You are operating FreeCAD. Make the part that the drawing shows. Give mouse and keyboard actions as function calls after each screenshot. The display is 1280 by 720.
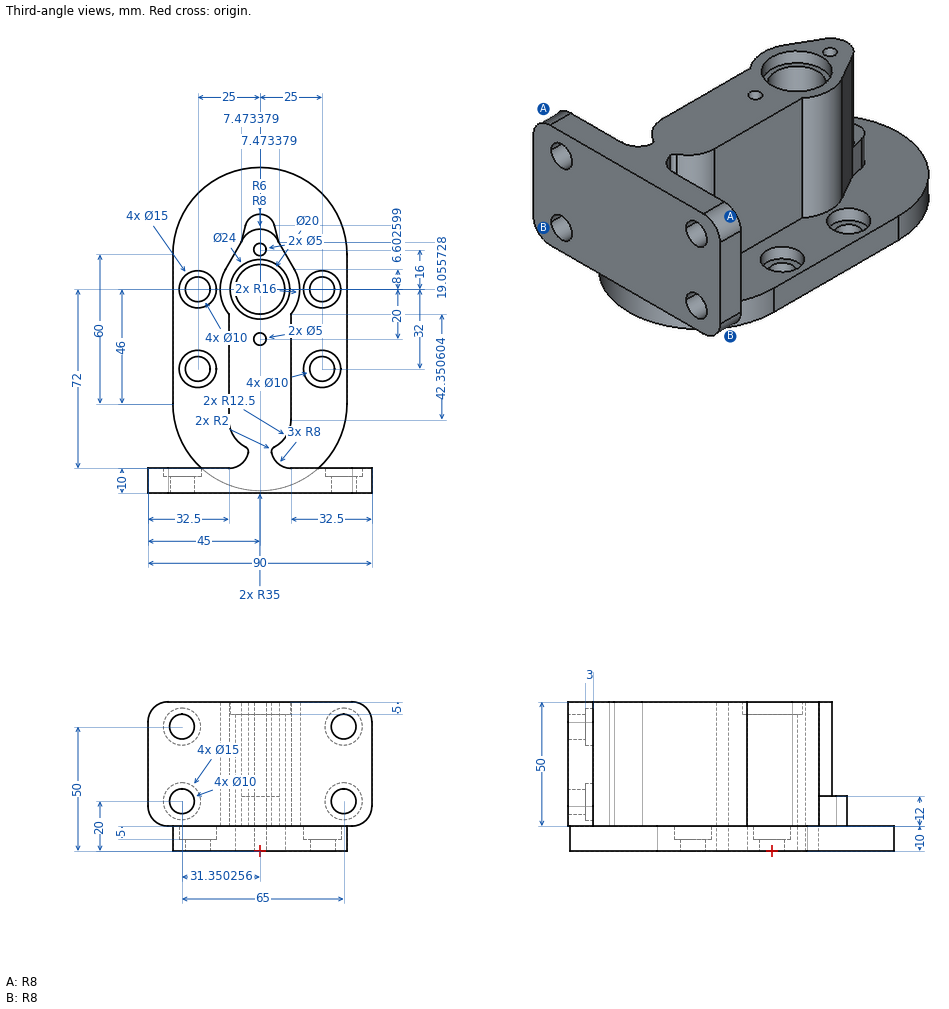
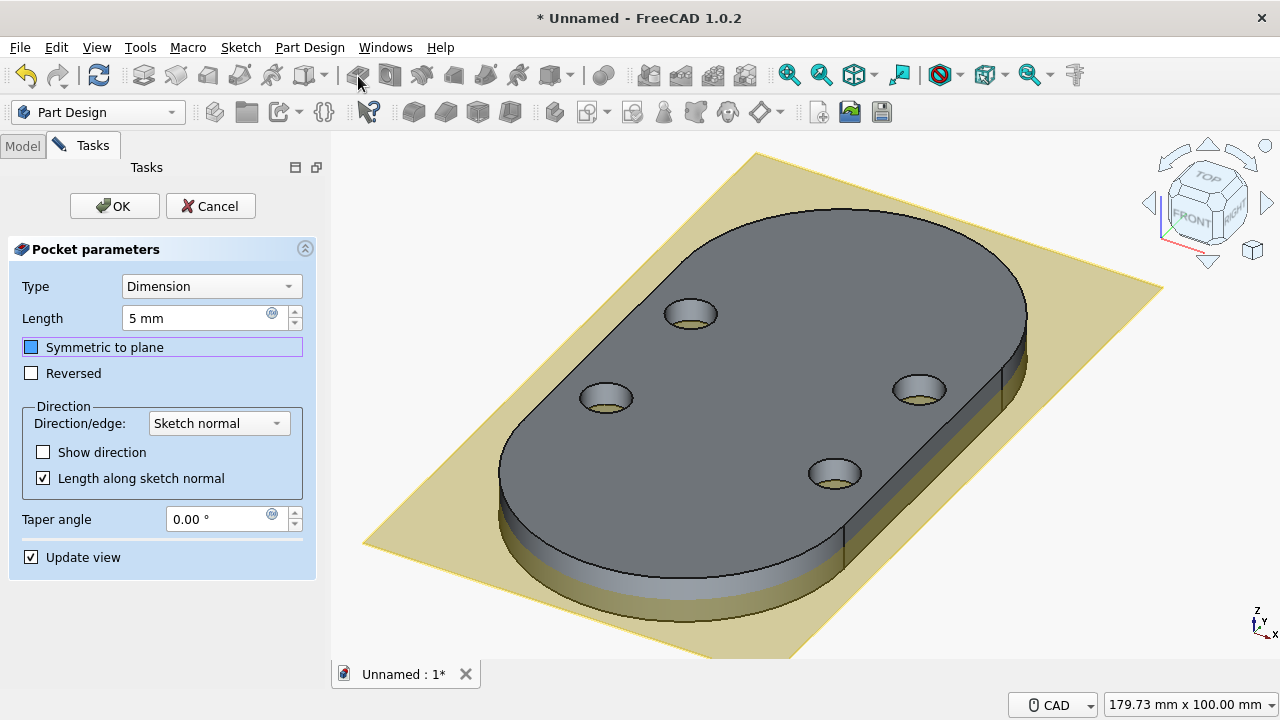
click(30, 373)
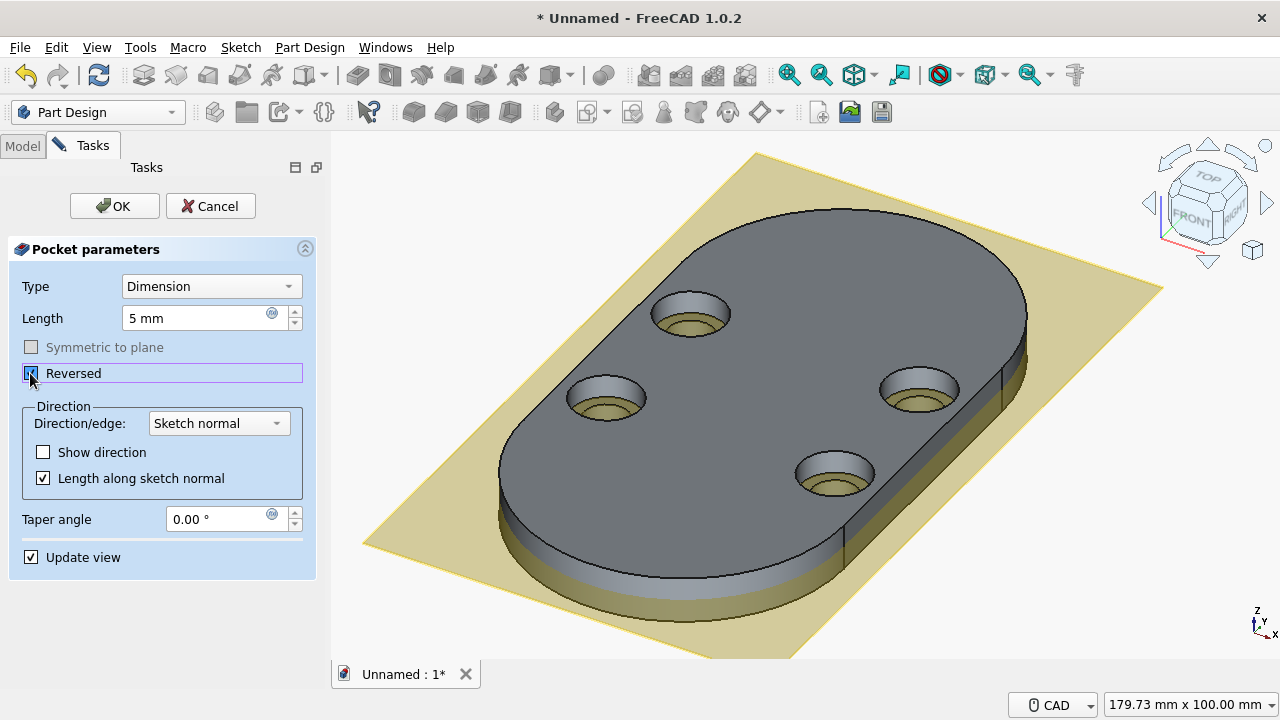
click(115, 206)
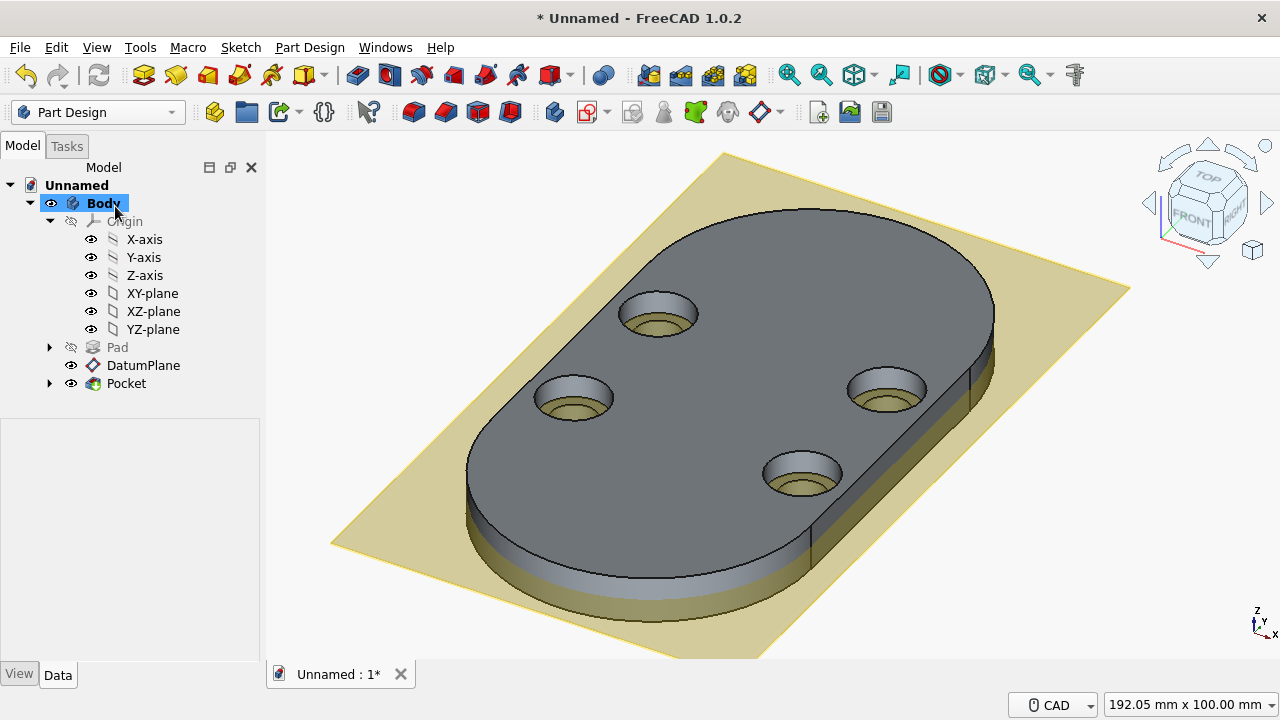
click(116, 365)
key(space)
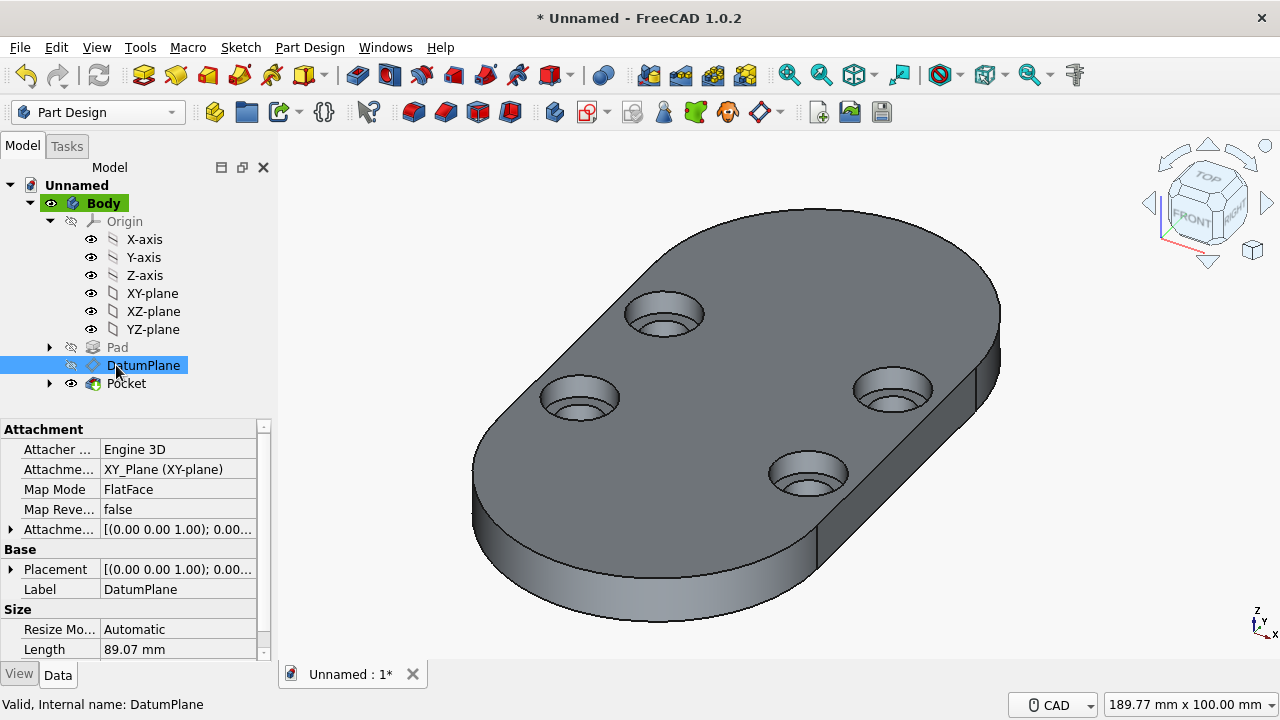
click(790, 76)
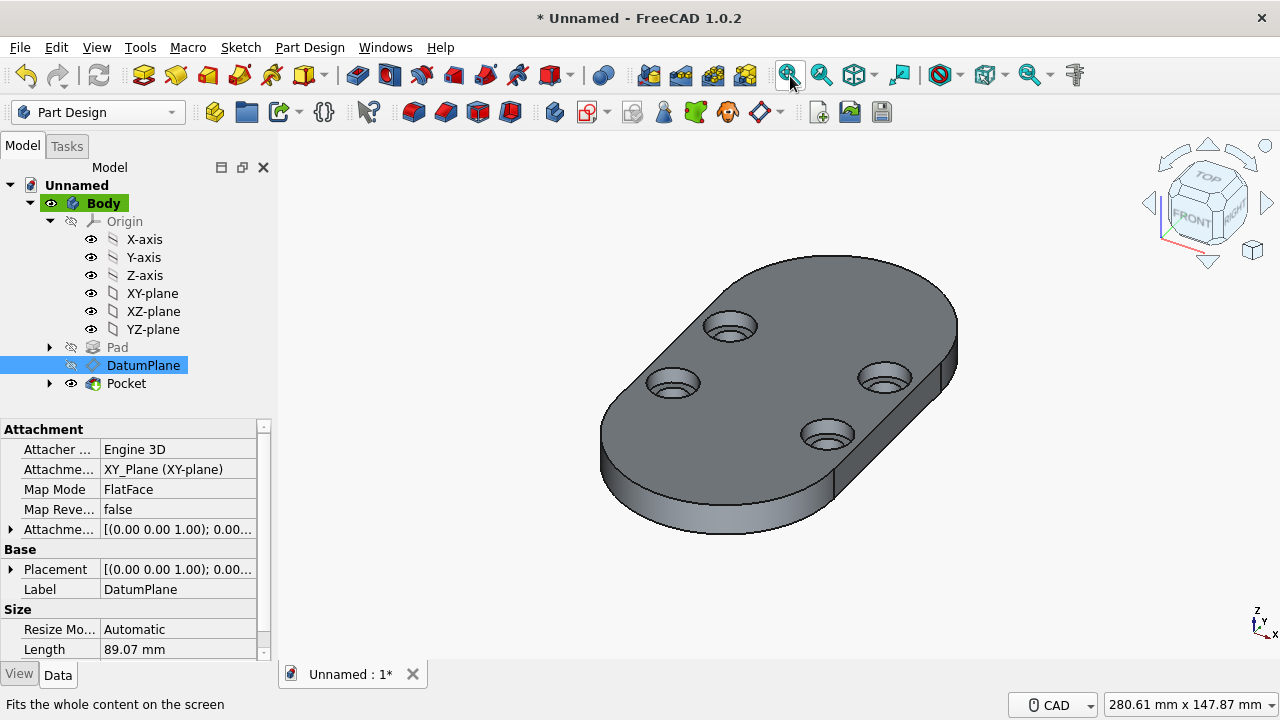
click(845, 313)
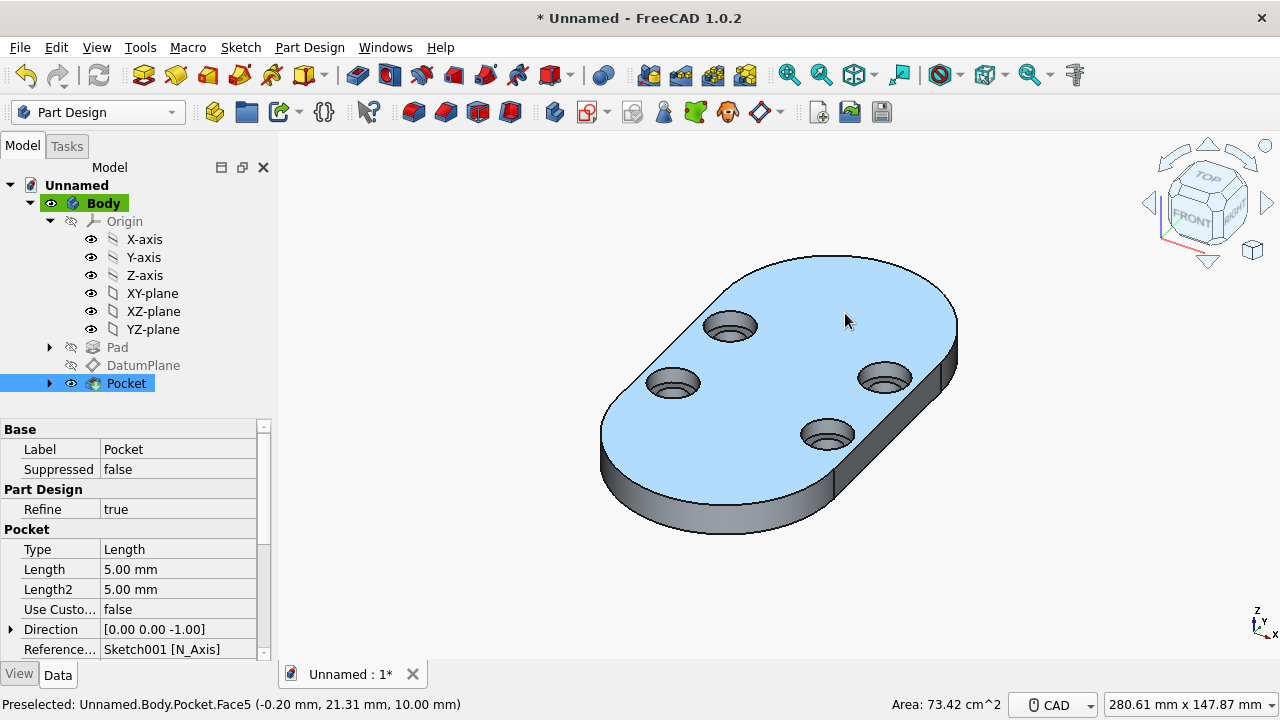
click(588, 112)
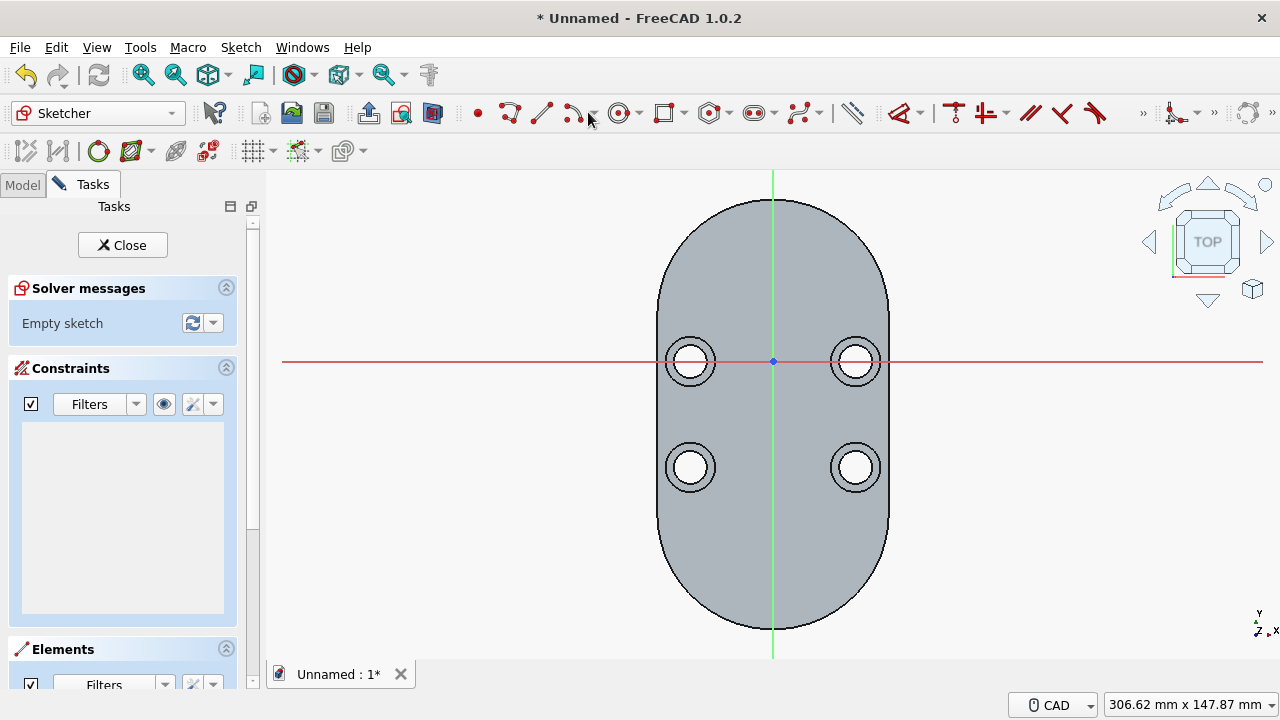
scroll(395, 222, down, 1)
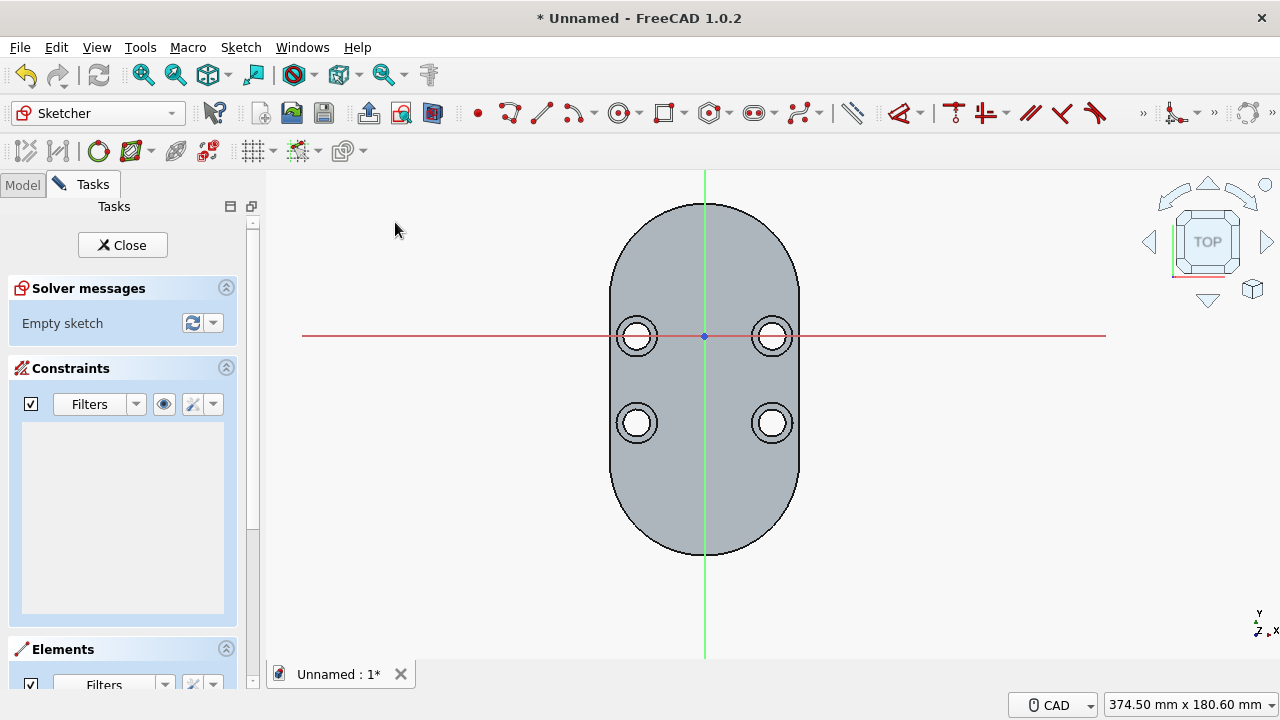
click(510, 114)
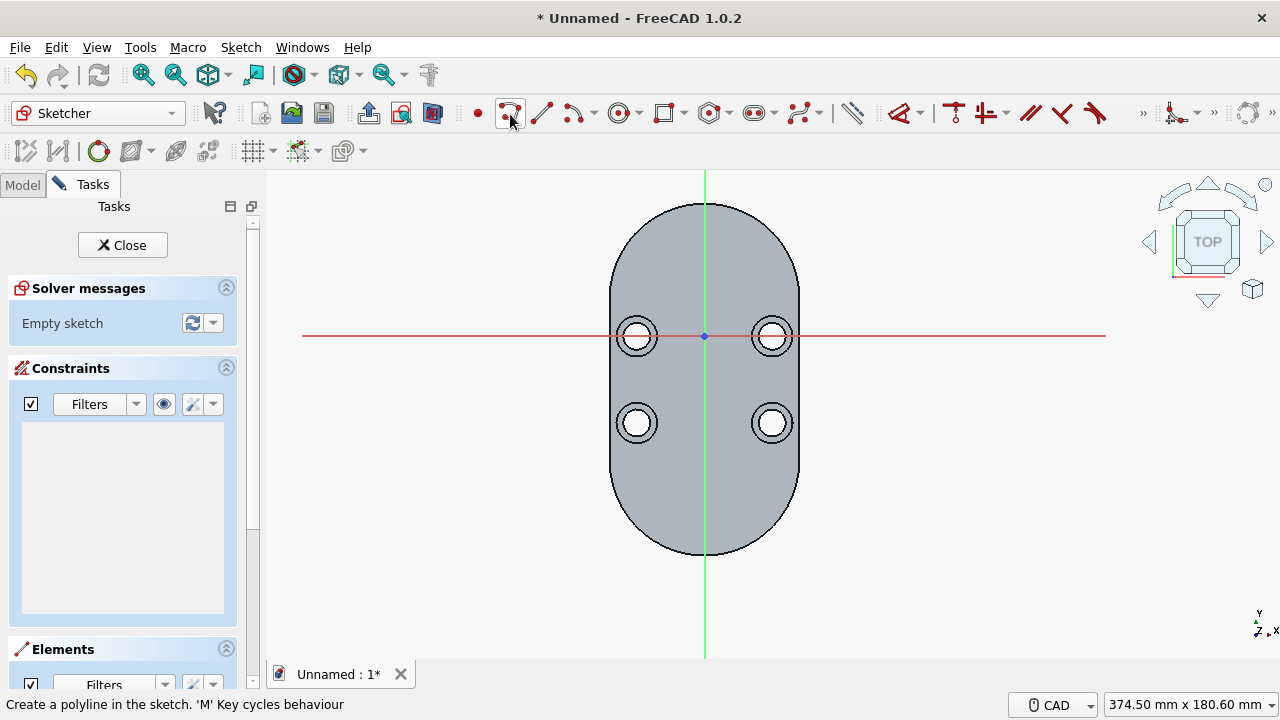
click(671, 531)
click(583, 531)
click(583, 558)
click(826, 558)
click(826, 531)
click(738, 531)
right_click(738, 531)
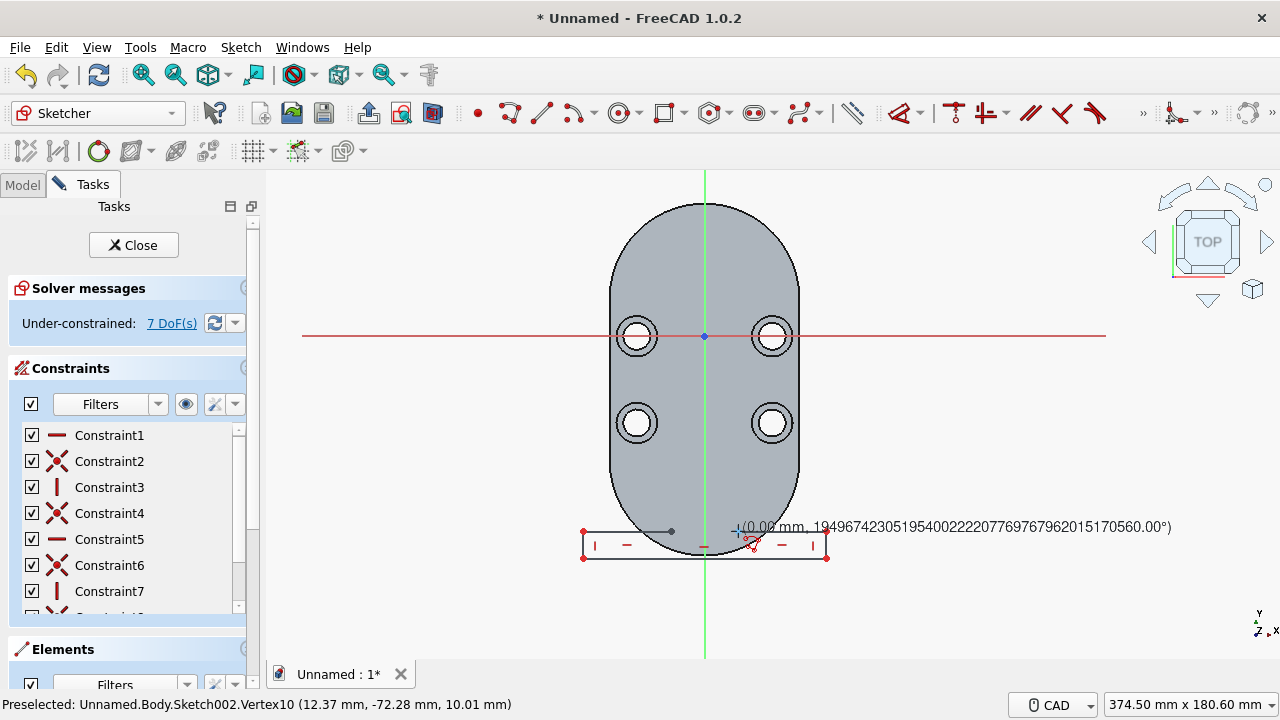
click(542, 114)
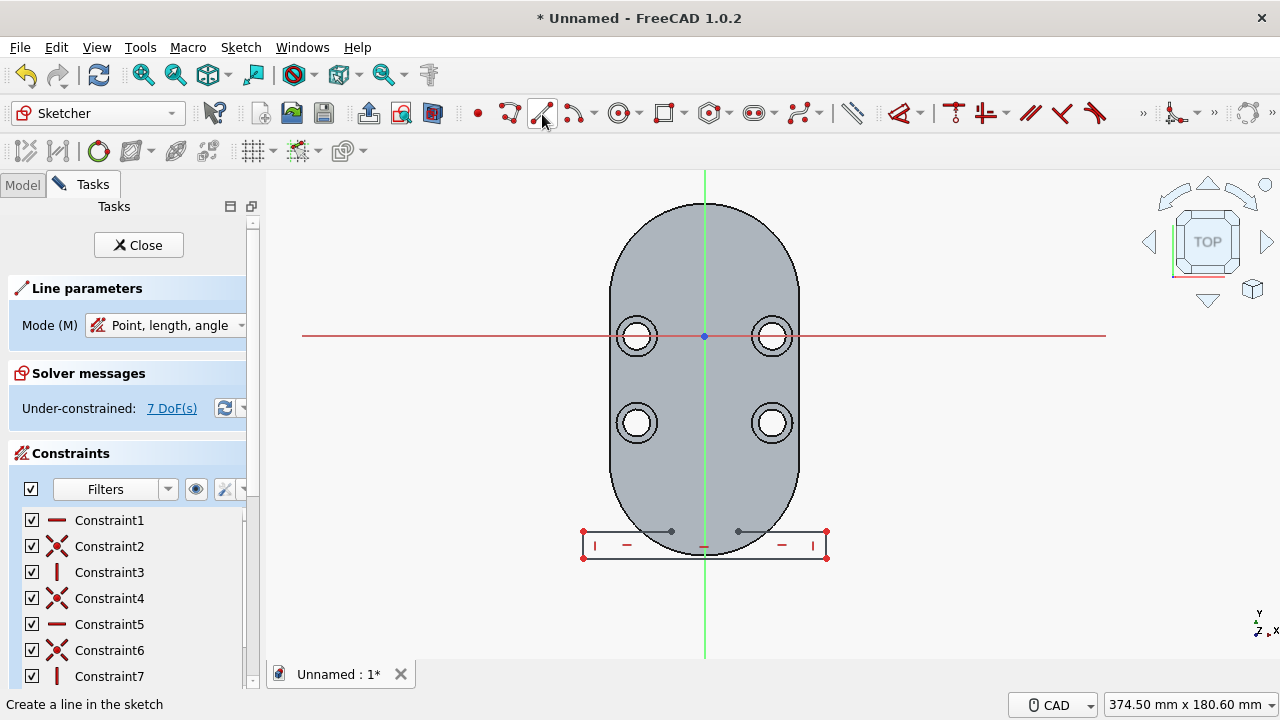
click(738, 478)
click(738, 363)